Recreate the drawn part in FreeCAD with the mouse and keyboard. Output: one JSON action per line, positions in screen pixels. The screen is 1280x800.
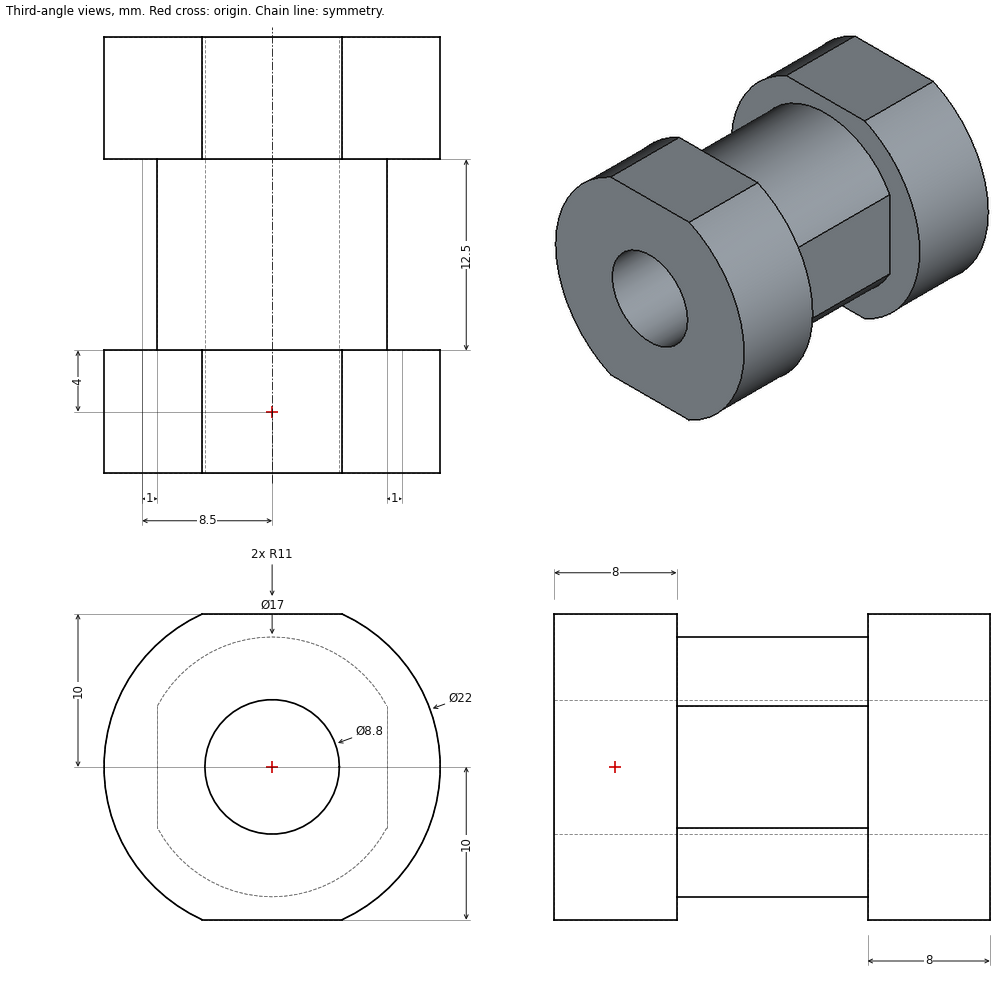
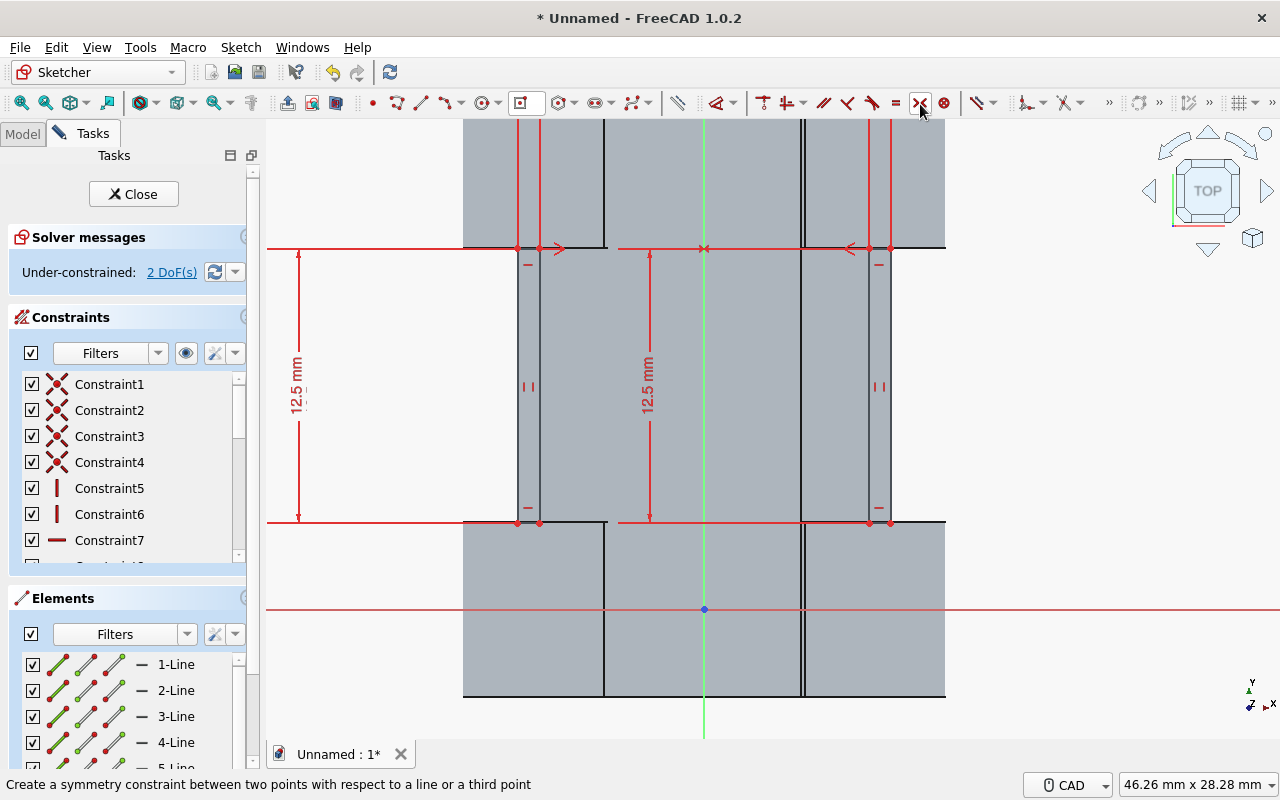
{"action": "left_click", "coordinate": [518, 523]}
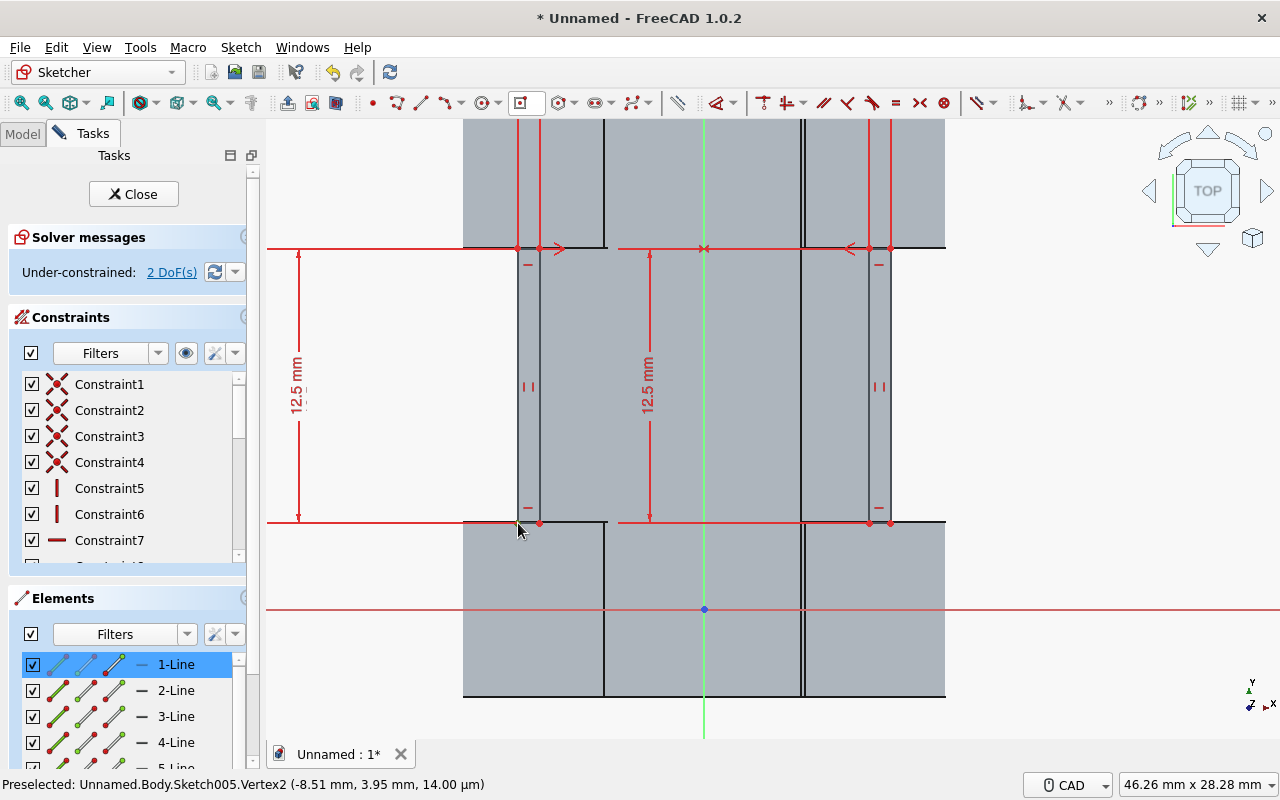
{"action": "left_click", "coordinate": [736, 104]}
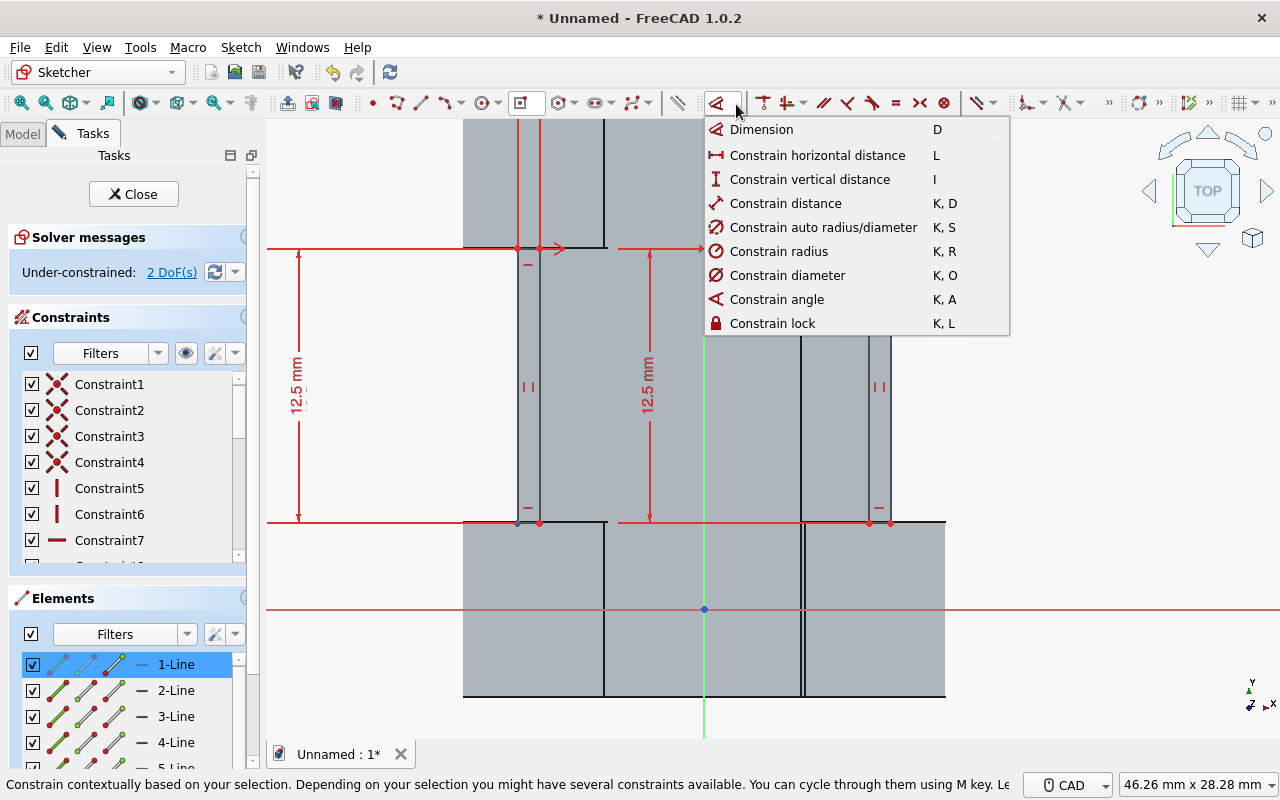
{"action": "left_click", "coordinate": [857, 179]}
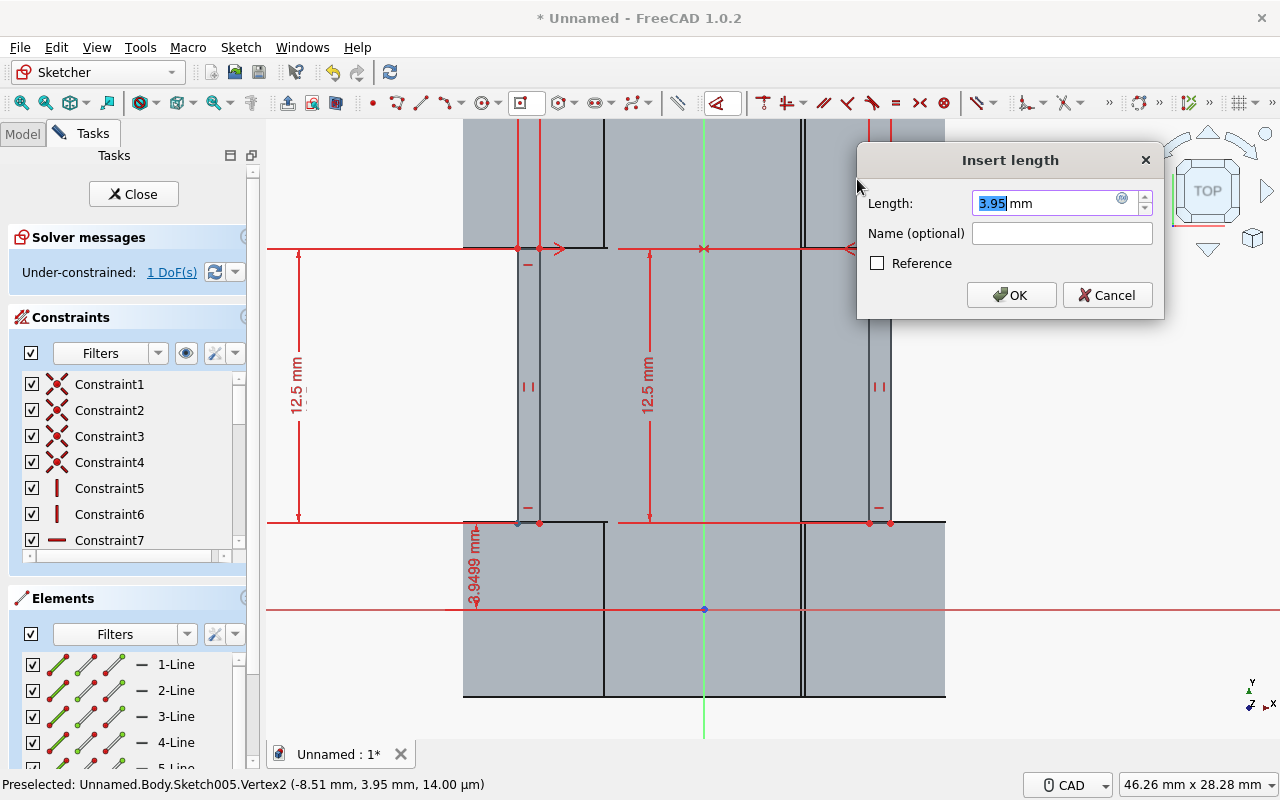
{"action": "type", "text": "4"}
{"action": "key", "text": "Return"}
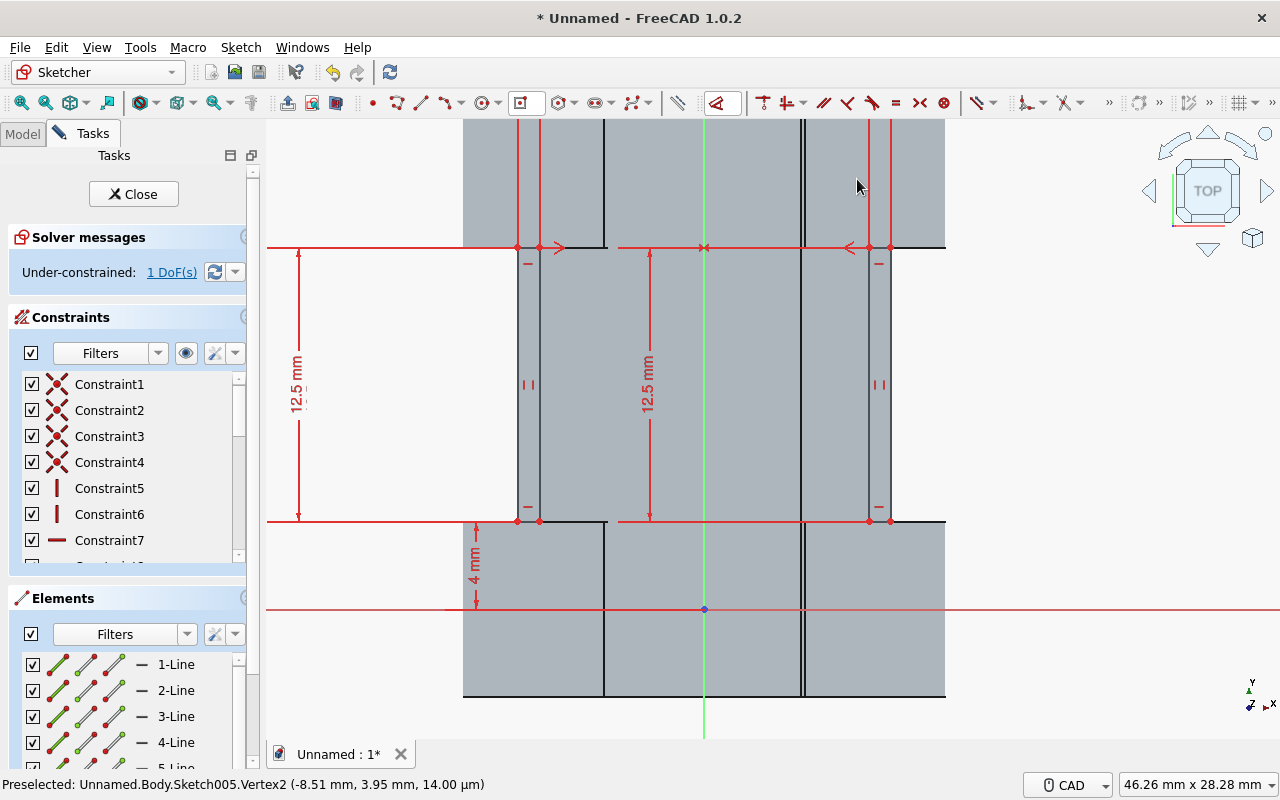
{"action": "left_click", "coordinate": [518, 248]}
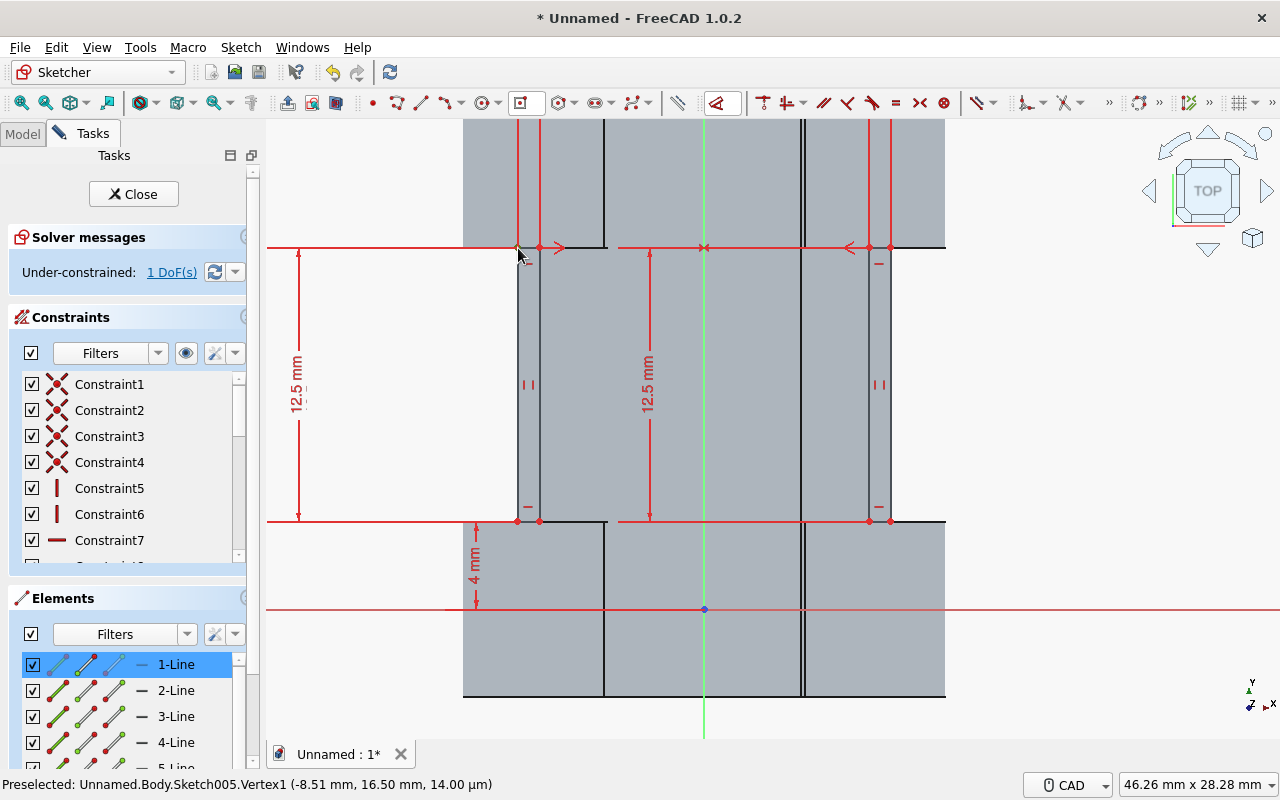
{"action": "key", "text": "l"}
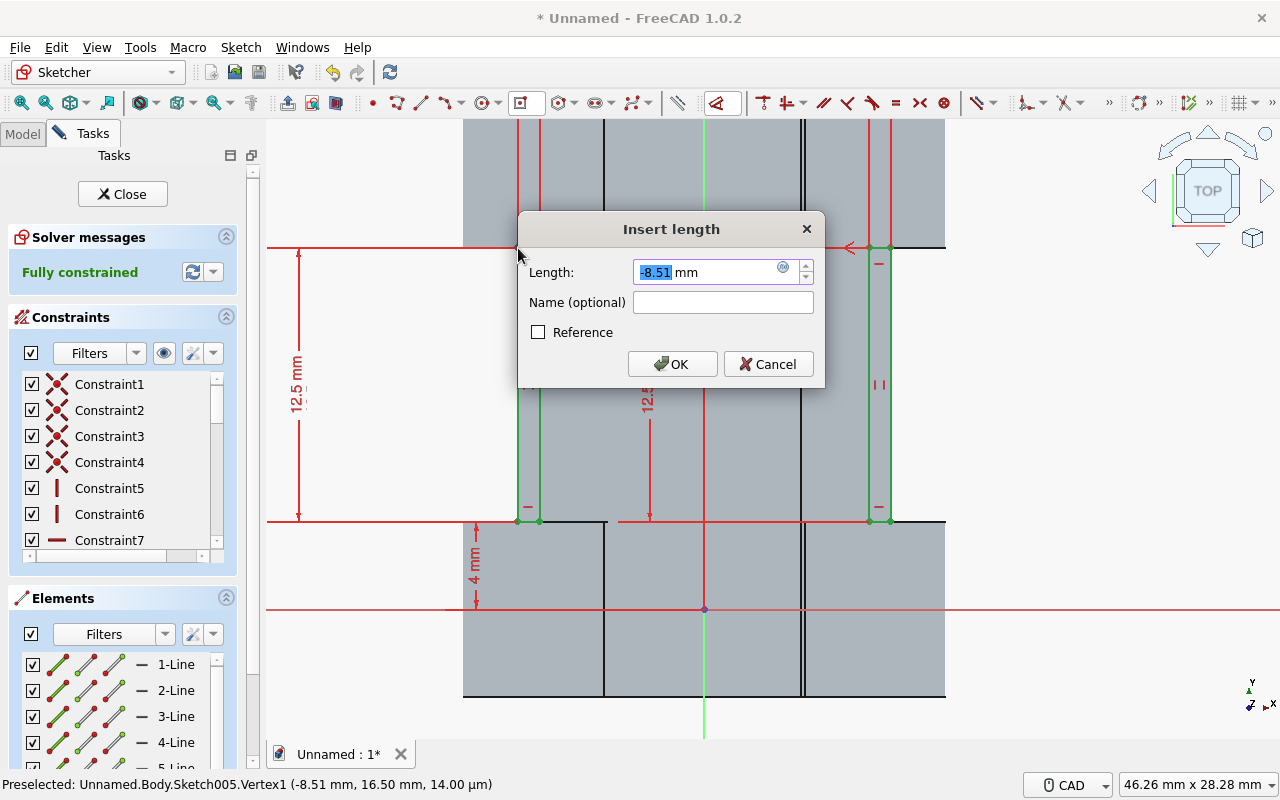
{"action": "type", "text": "-8.5"}
{"action": "key", "text": "Return"}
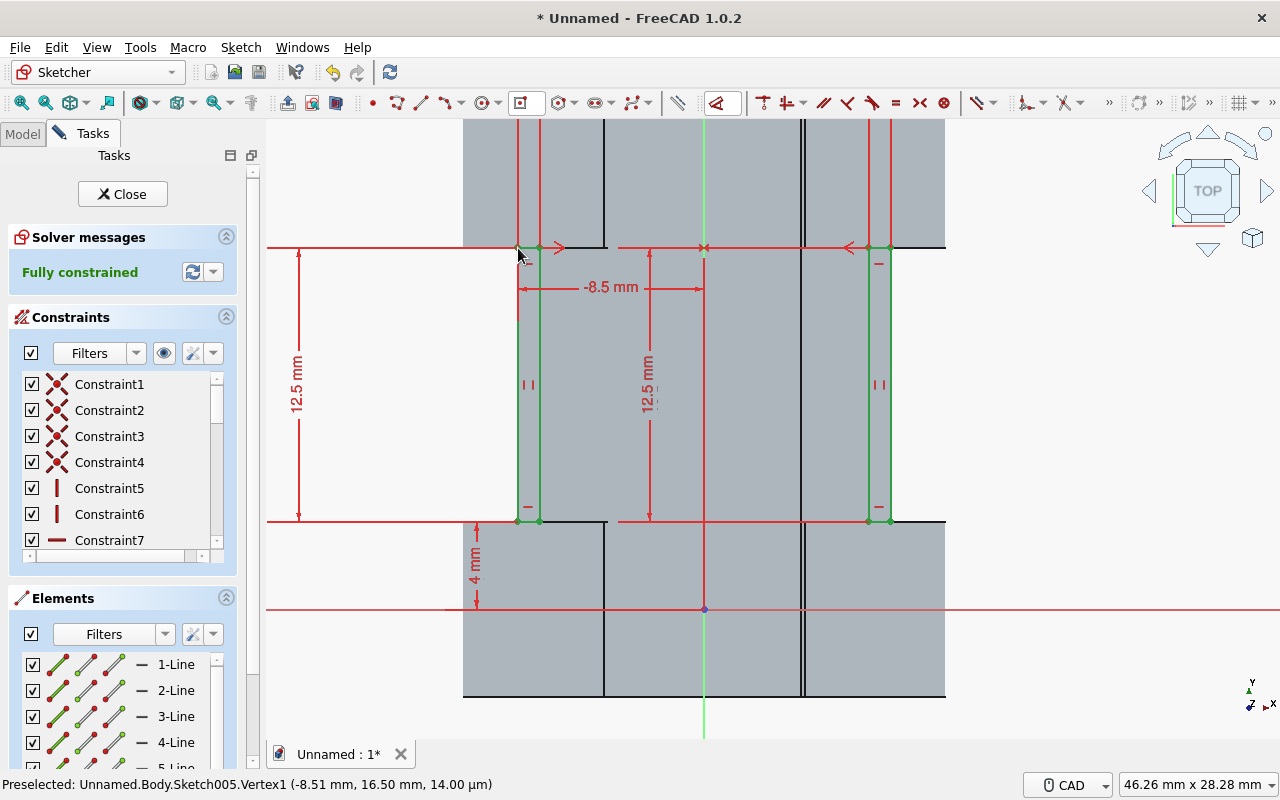
{"action": "left_click", "coordinate": [123, 194]}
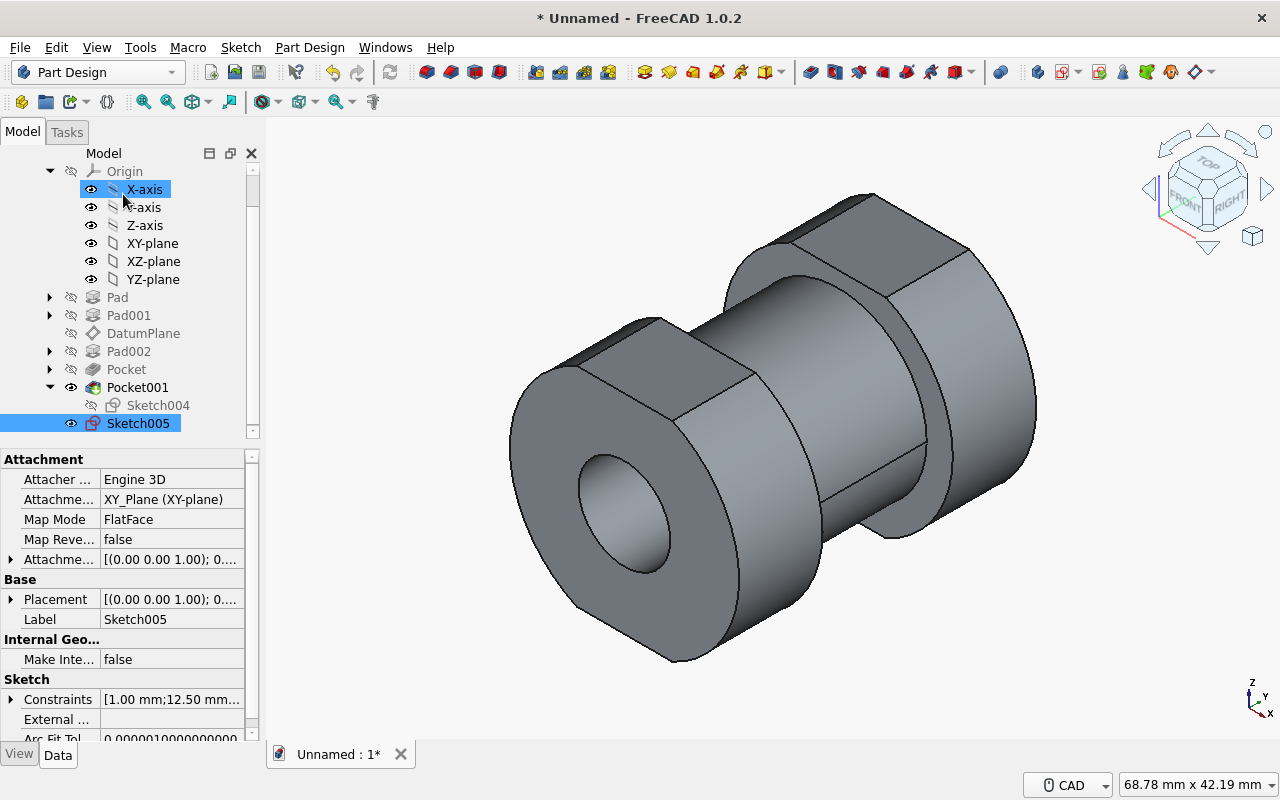
{"action": "left_click", "coordinate": [812, 72]}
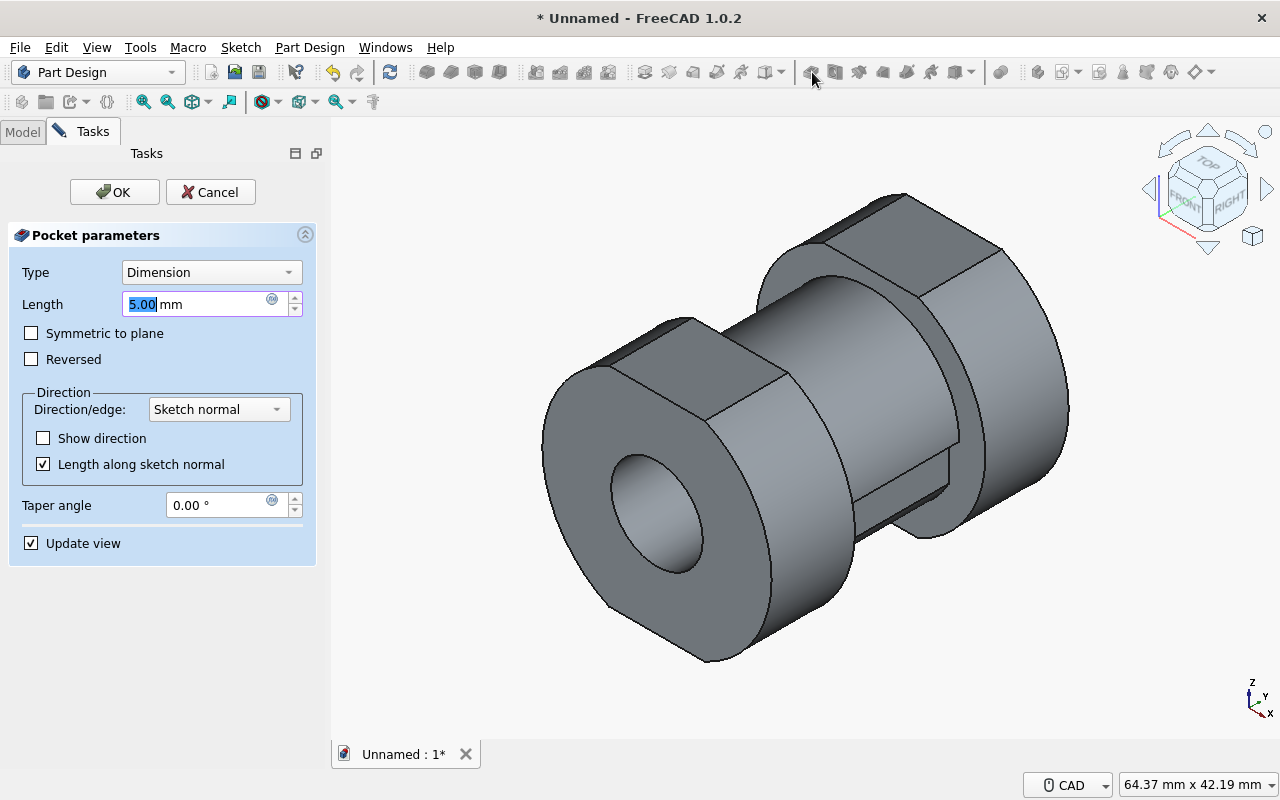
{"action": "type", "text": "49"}
{"action": "key", "text": "Tab"}